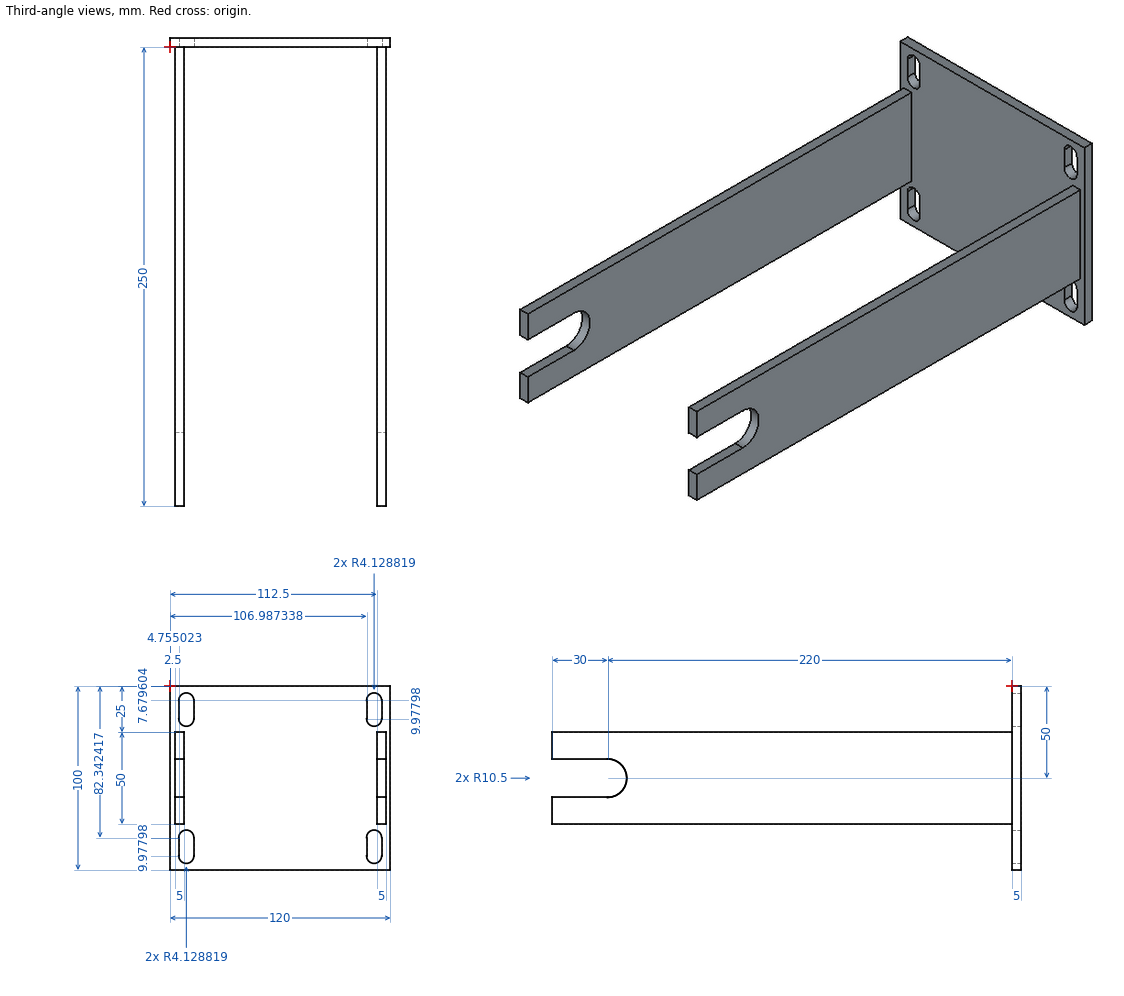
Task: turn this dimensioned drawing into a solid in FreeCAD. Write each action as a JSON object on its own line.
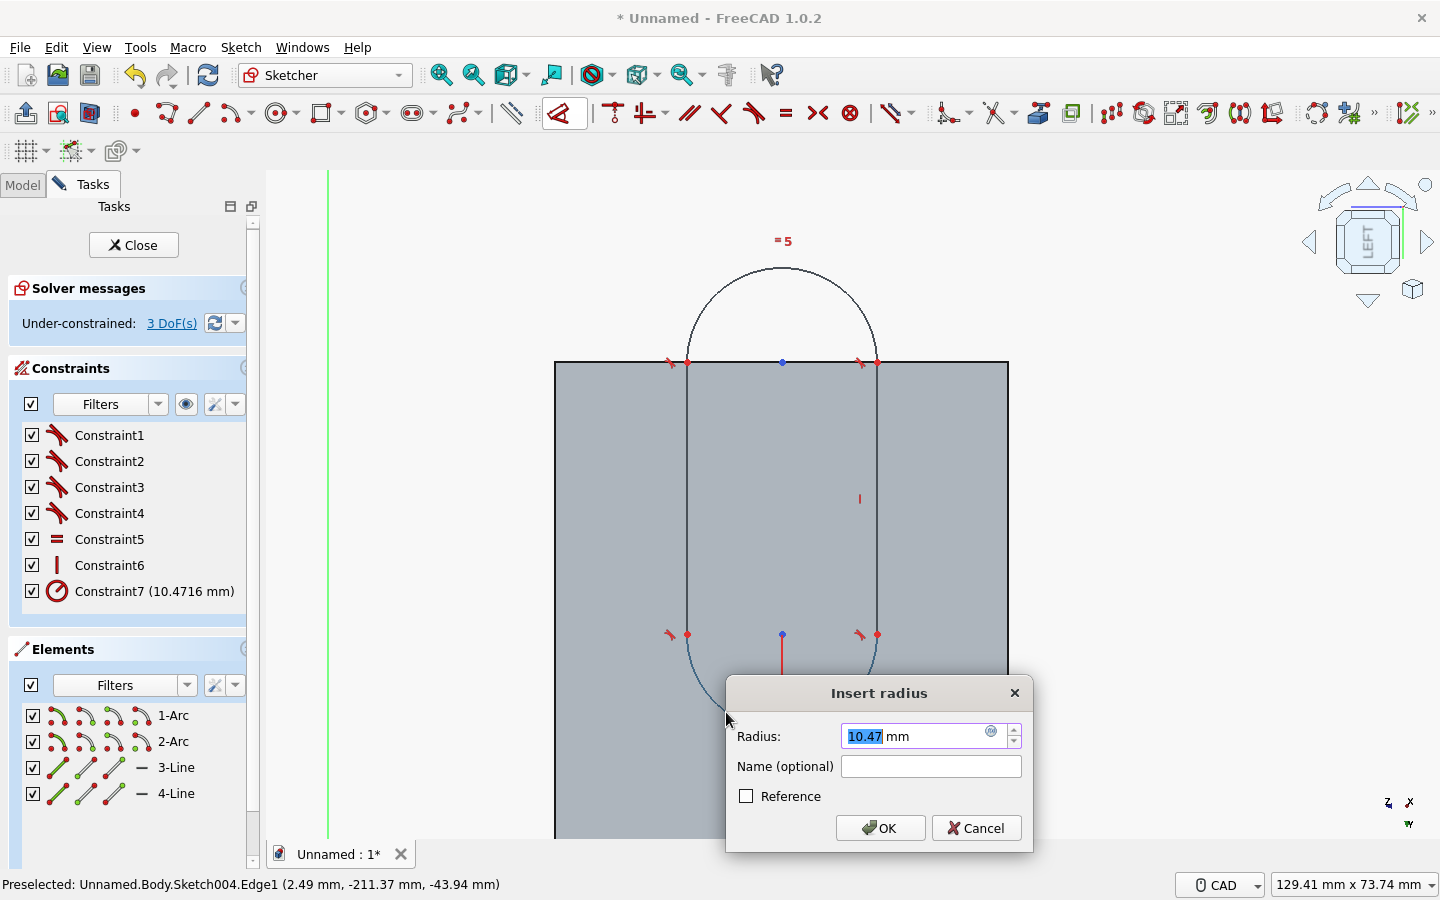
{"action": "type", "text": "10.5"}
{"action": "key", "text": "Return"}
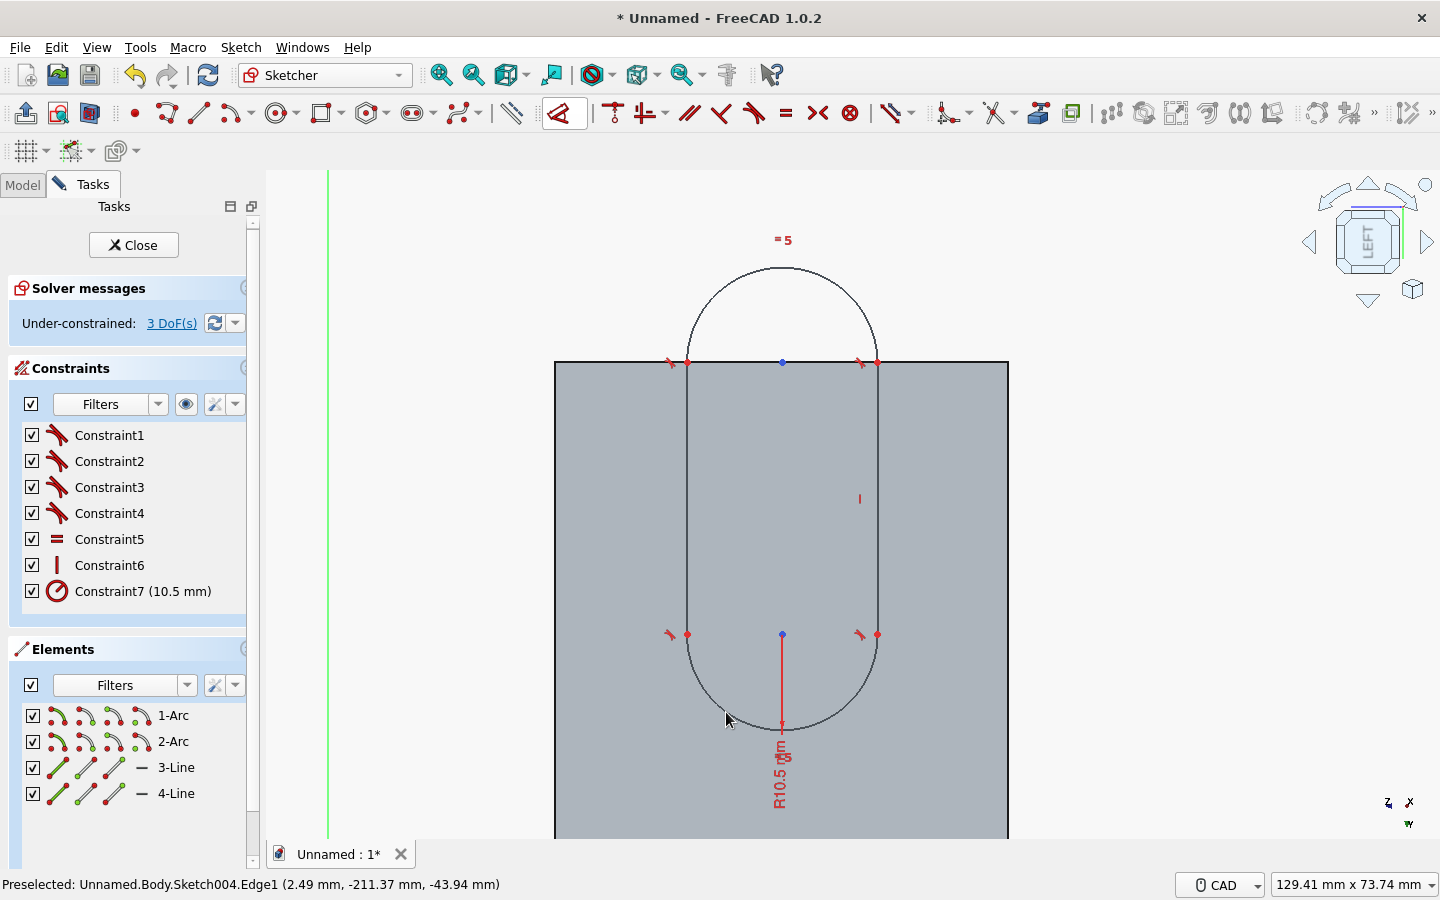
{"action": "left_click", "coordinate": [687, 553]}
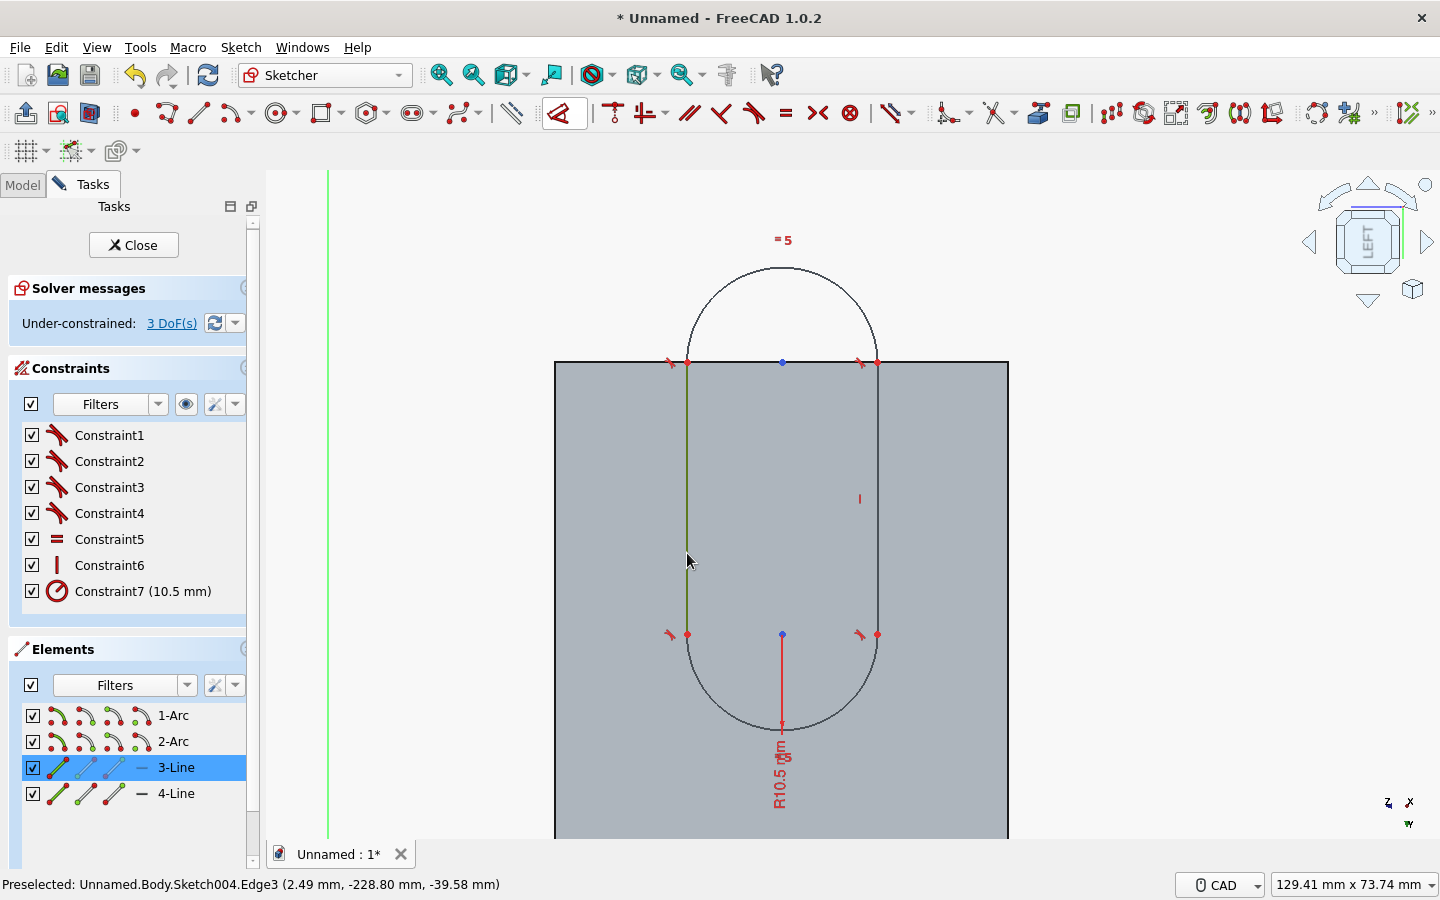
{"action": "key", "text": "i"}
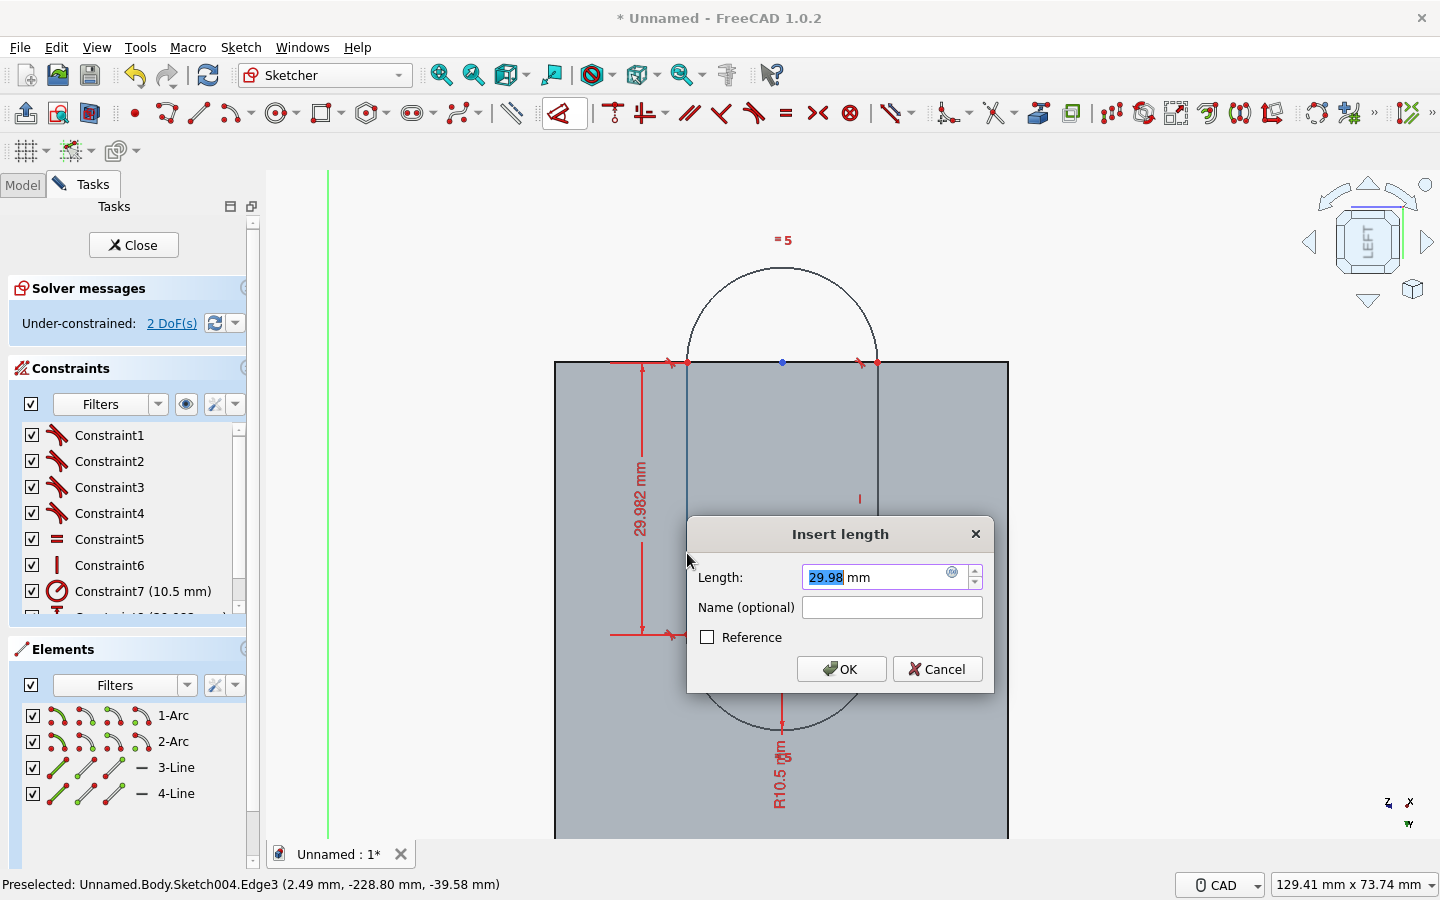
{"action": "type", "text": "30"}
{"action": "key", "text": "Return"}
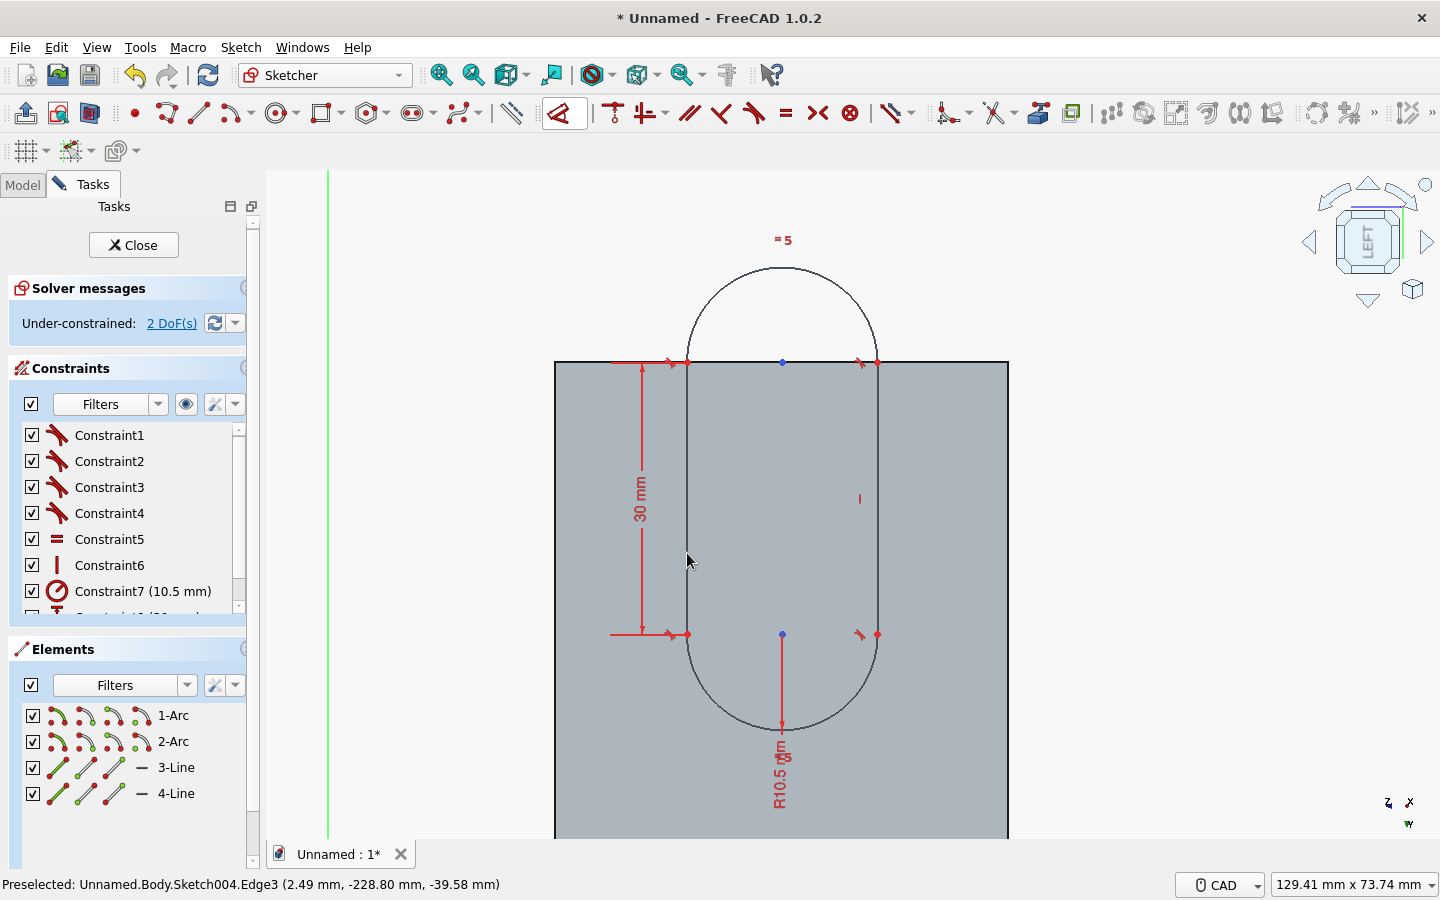
{"action": "left_click", "coordinate": [782, 635]}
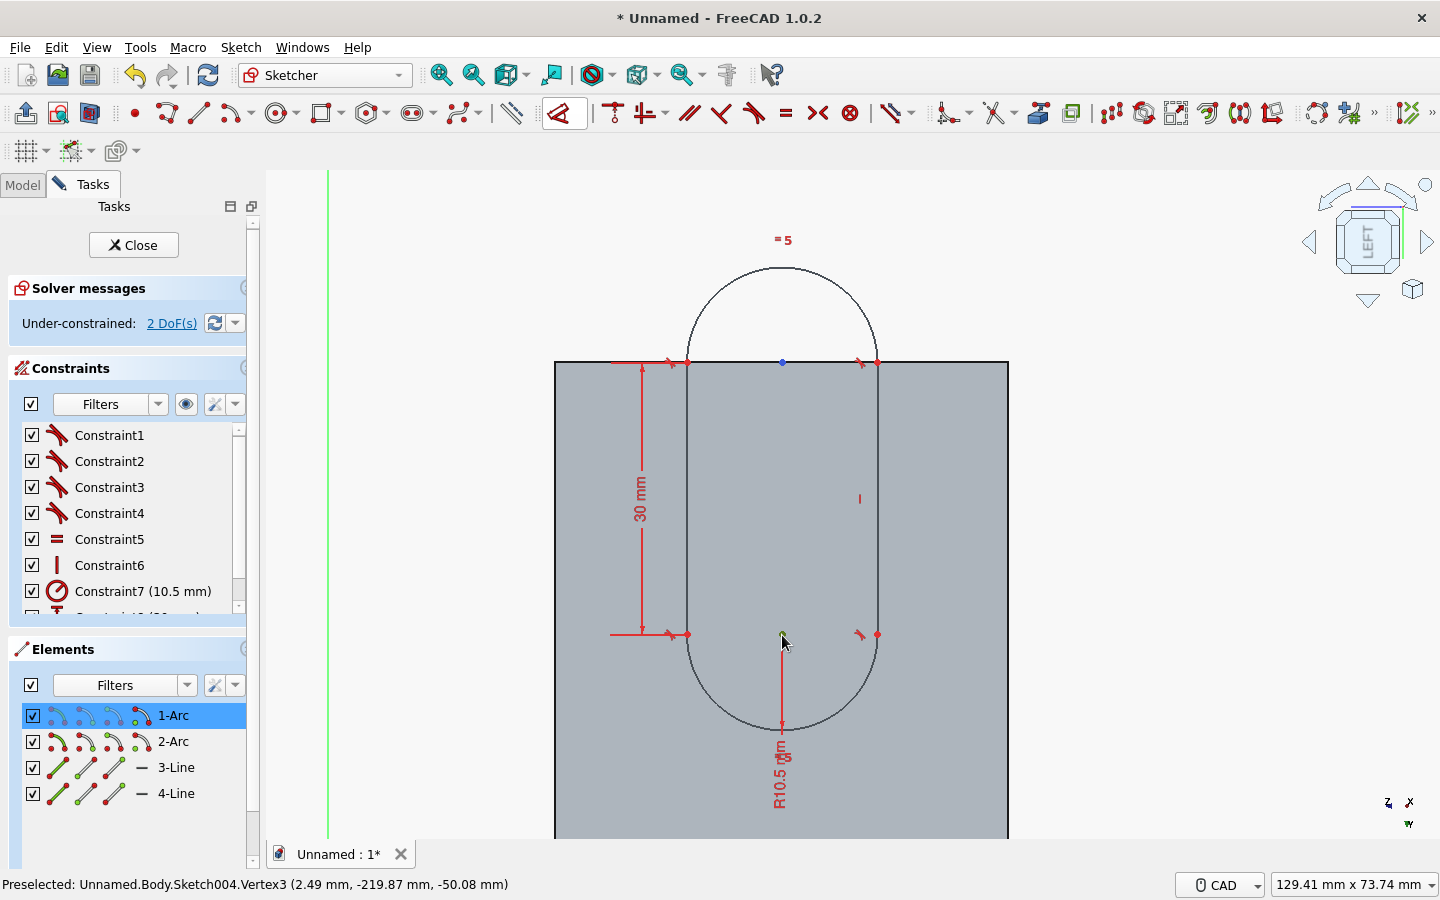
{"action": "left_click", "coordinate": [582, 114]}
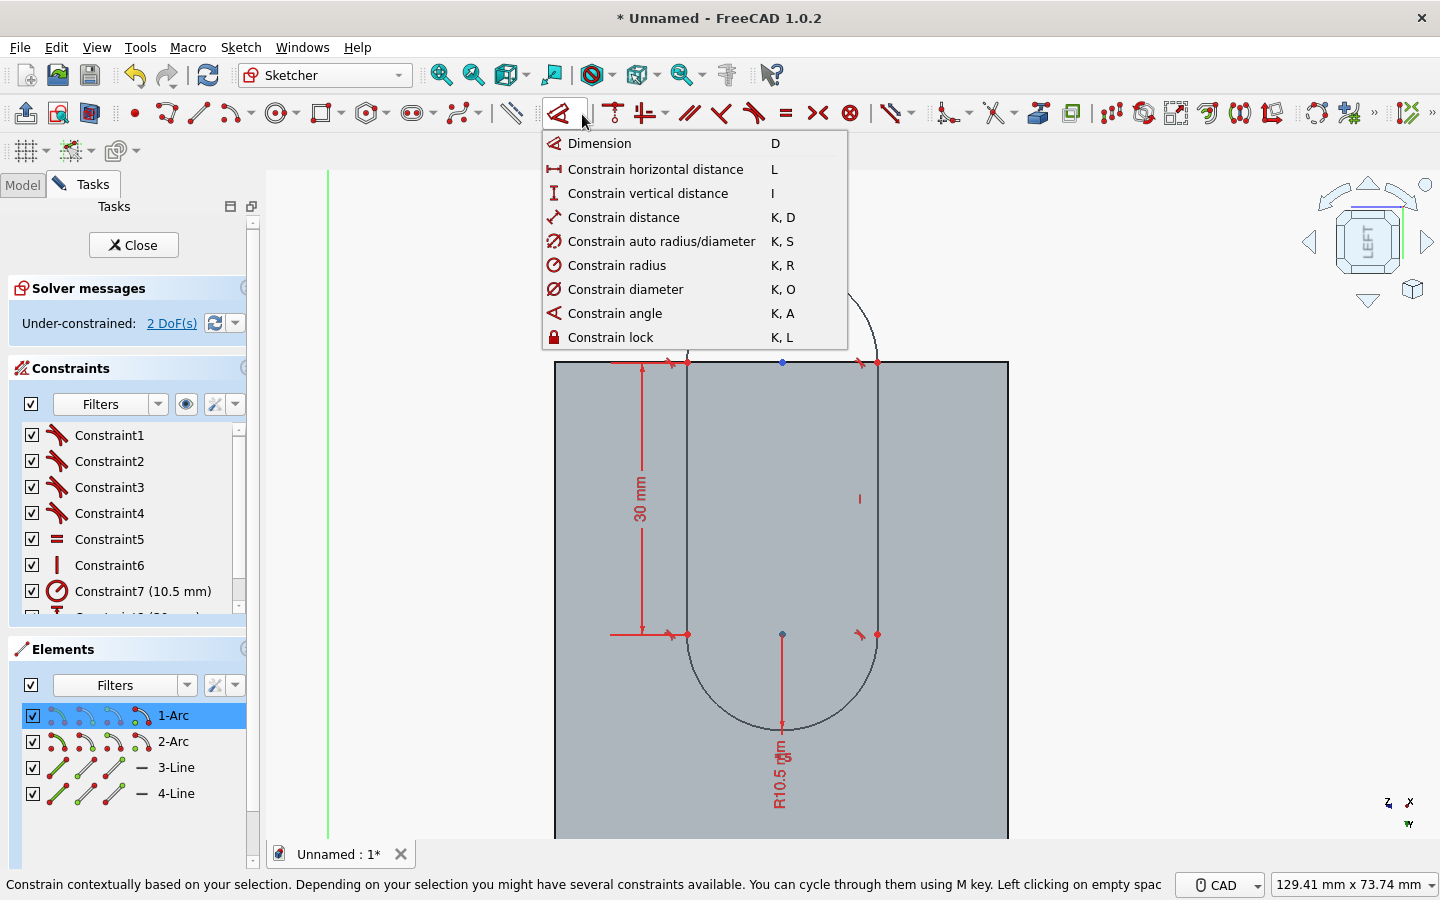
{"action": "left_click", "coordinate": [695, 169]}